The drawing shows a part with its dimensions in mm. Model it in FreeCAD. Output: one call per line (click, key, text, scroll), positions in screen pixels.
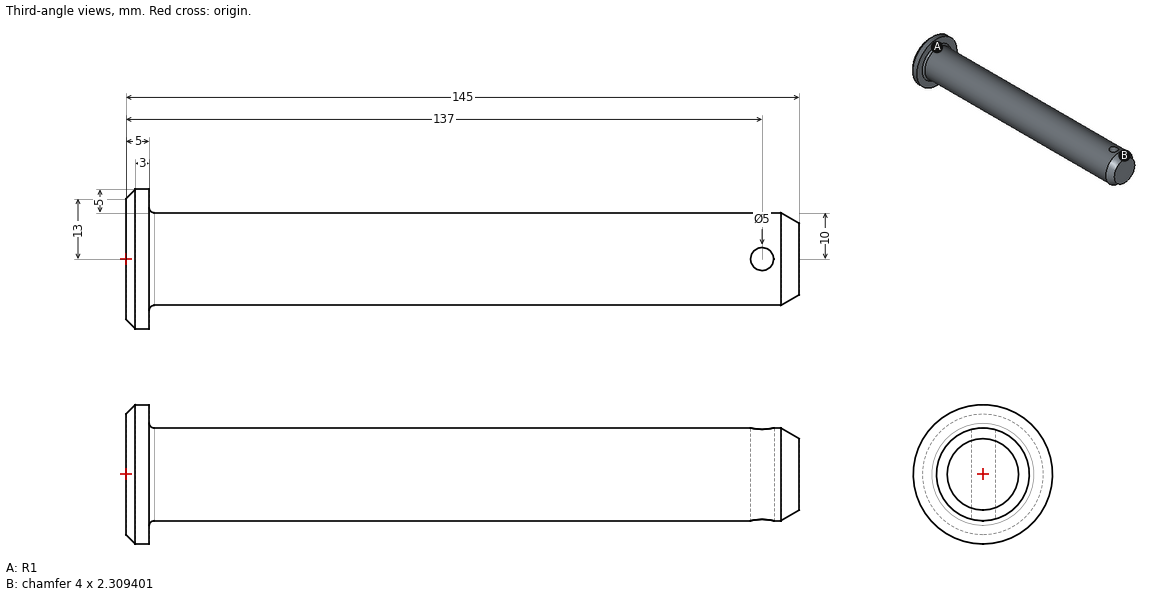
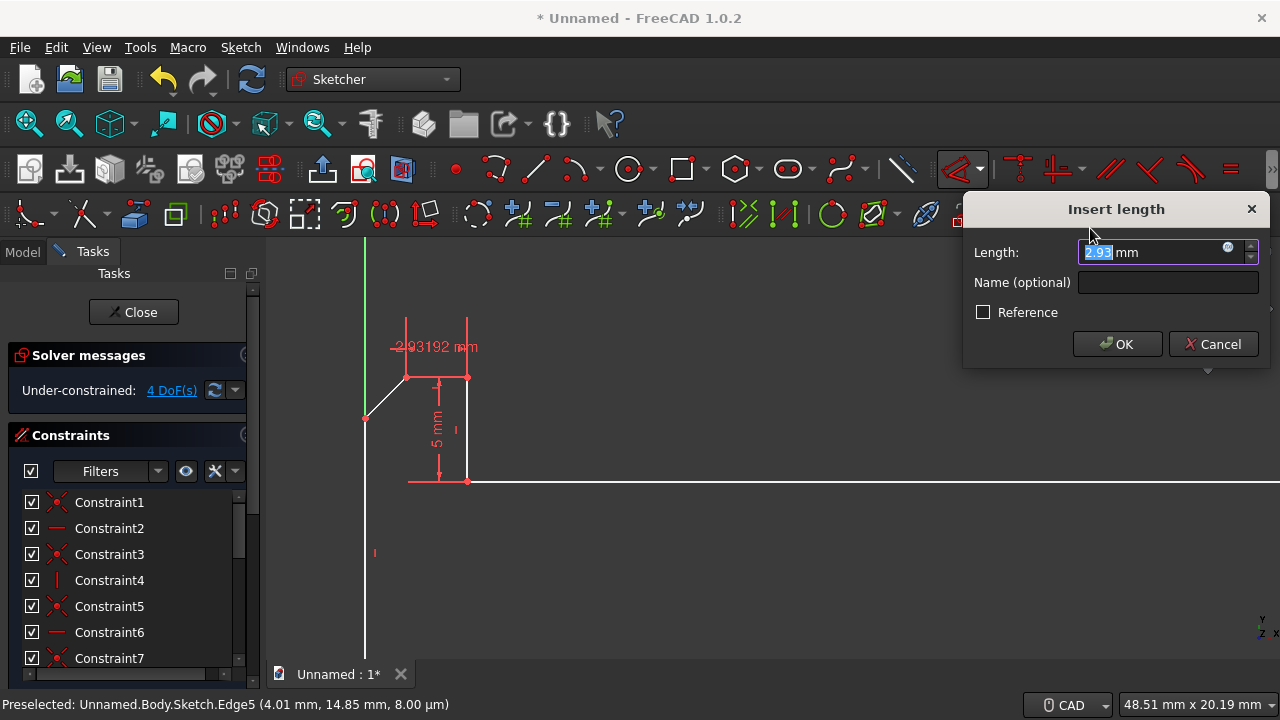
text(3)
key(Return)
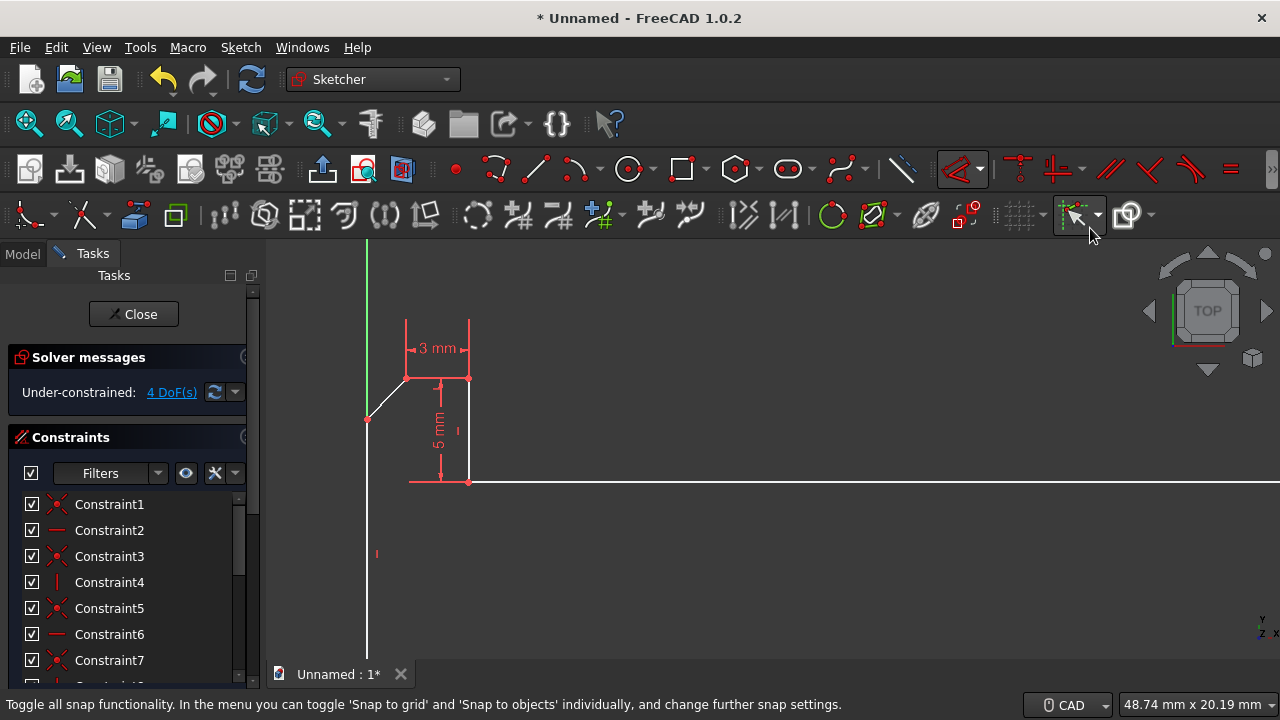
scroll(408, 428, down, 8)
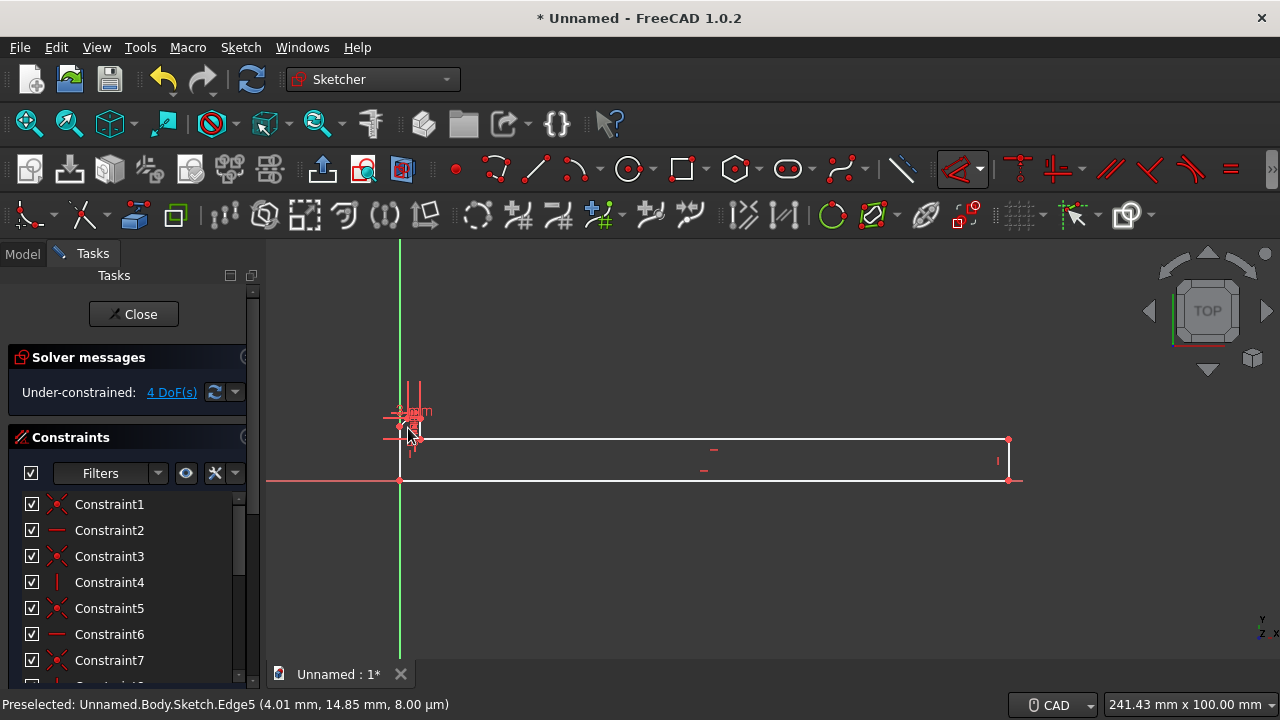
click(1009, 468)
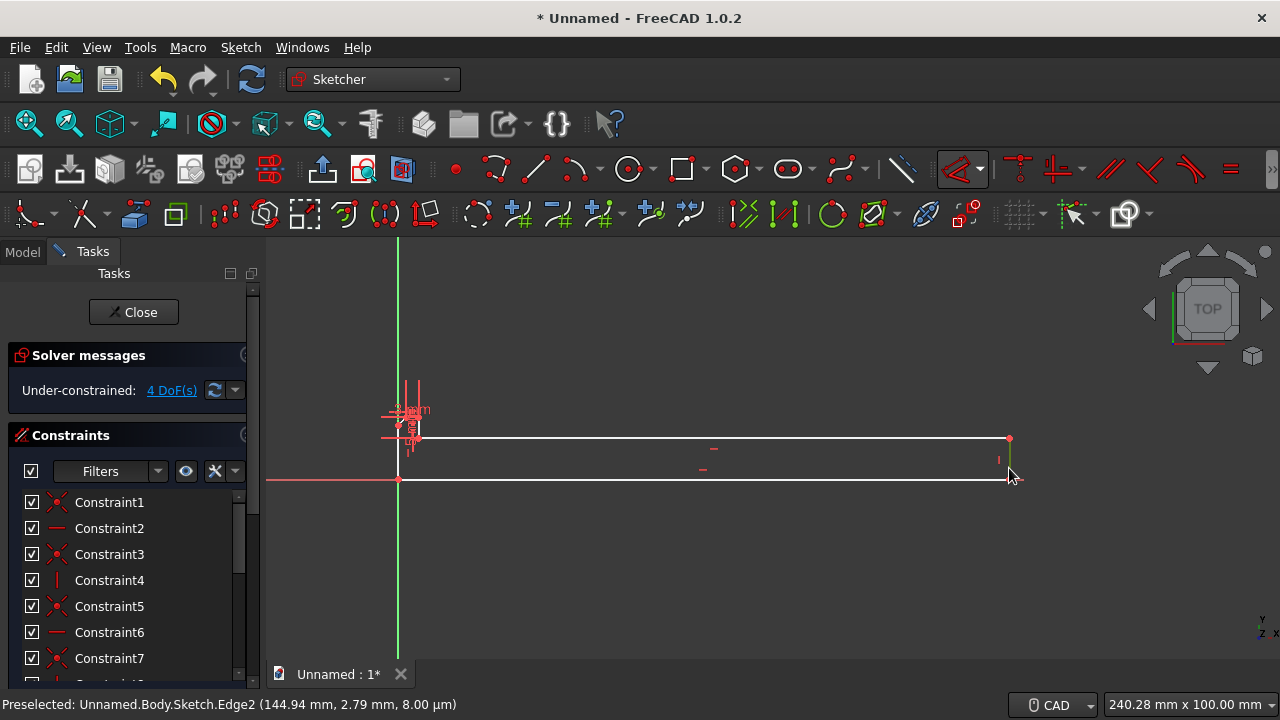
key(i)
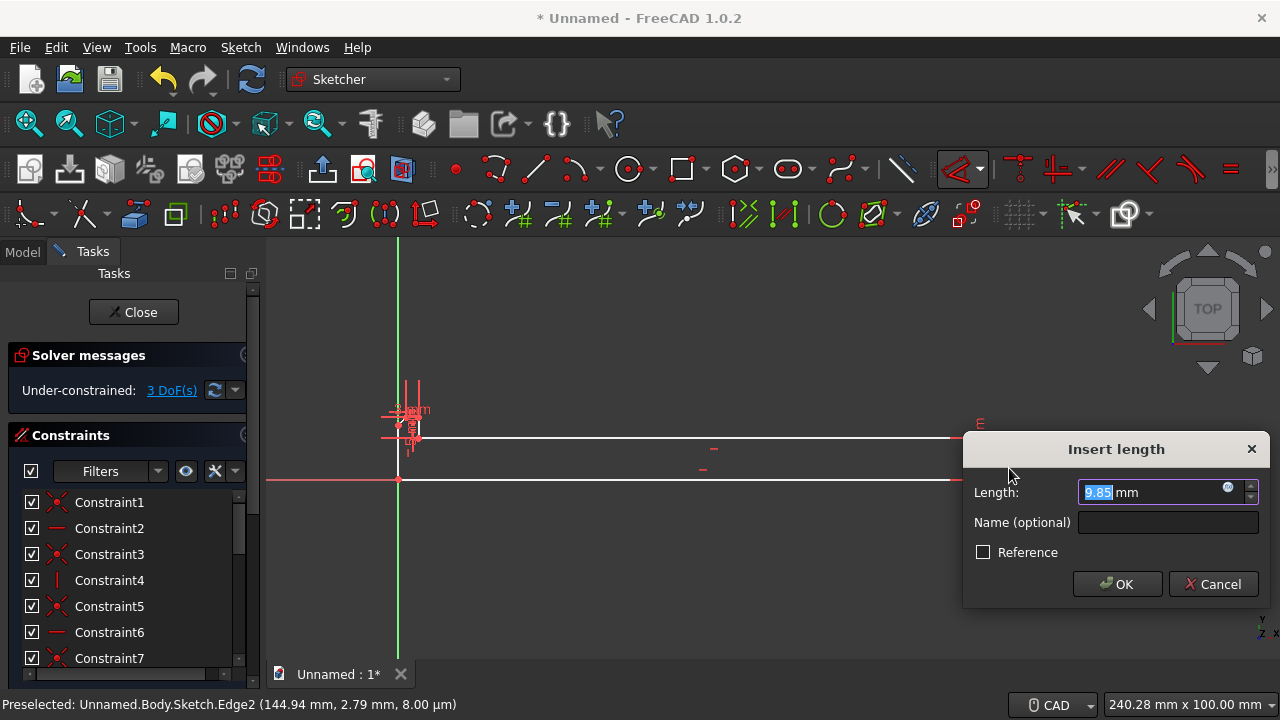
text(10)
key(Return)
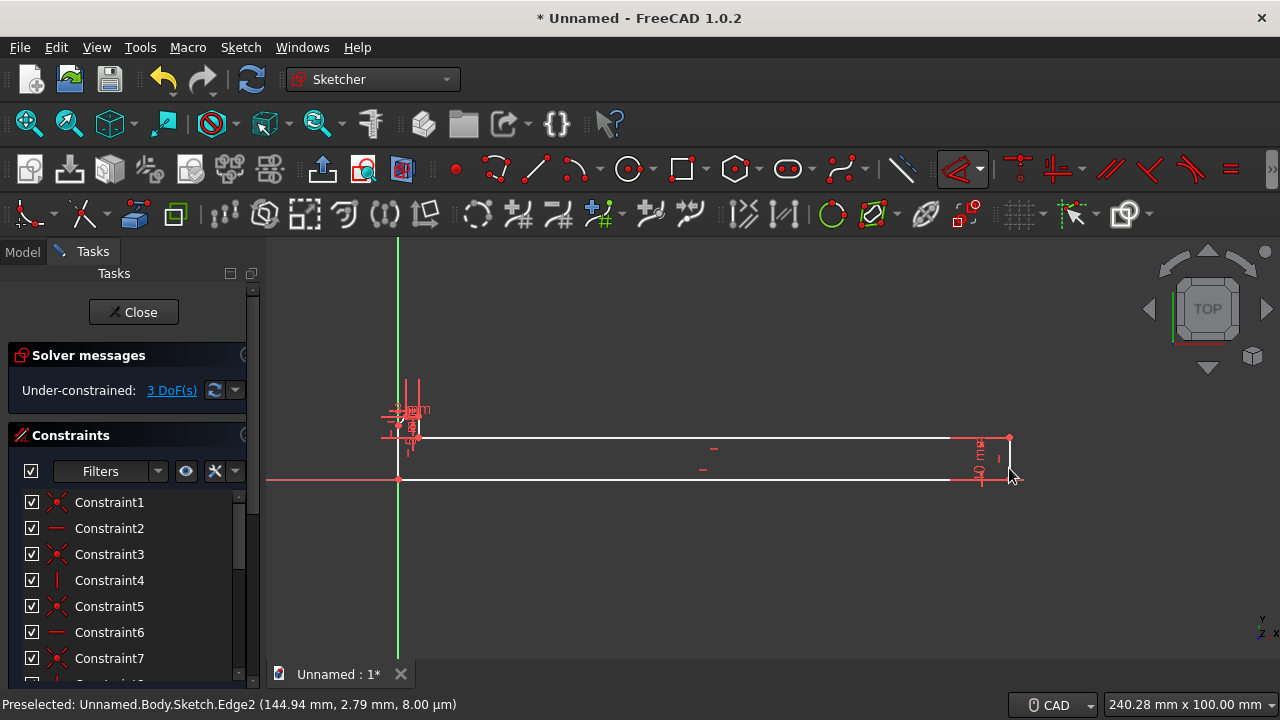
click(398, 442)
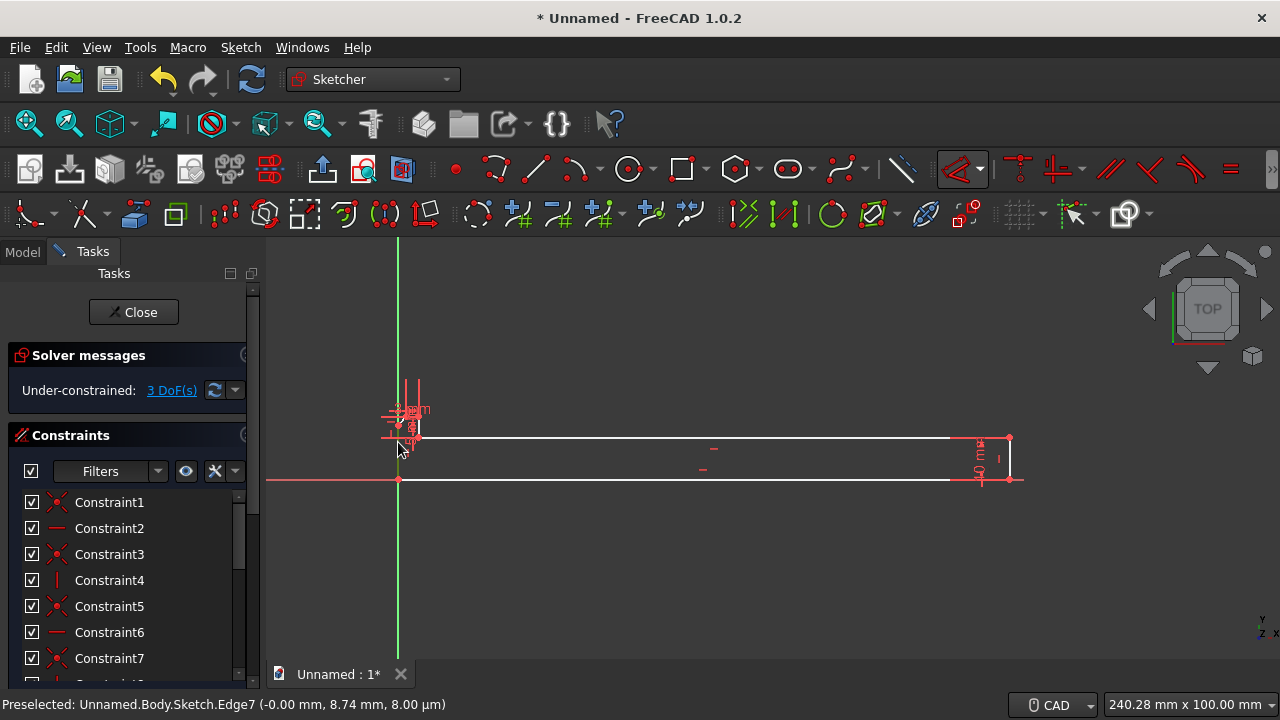
key(i)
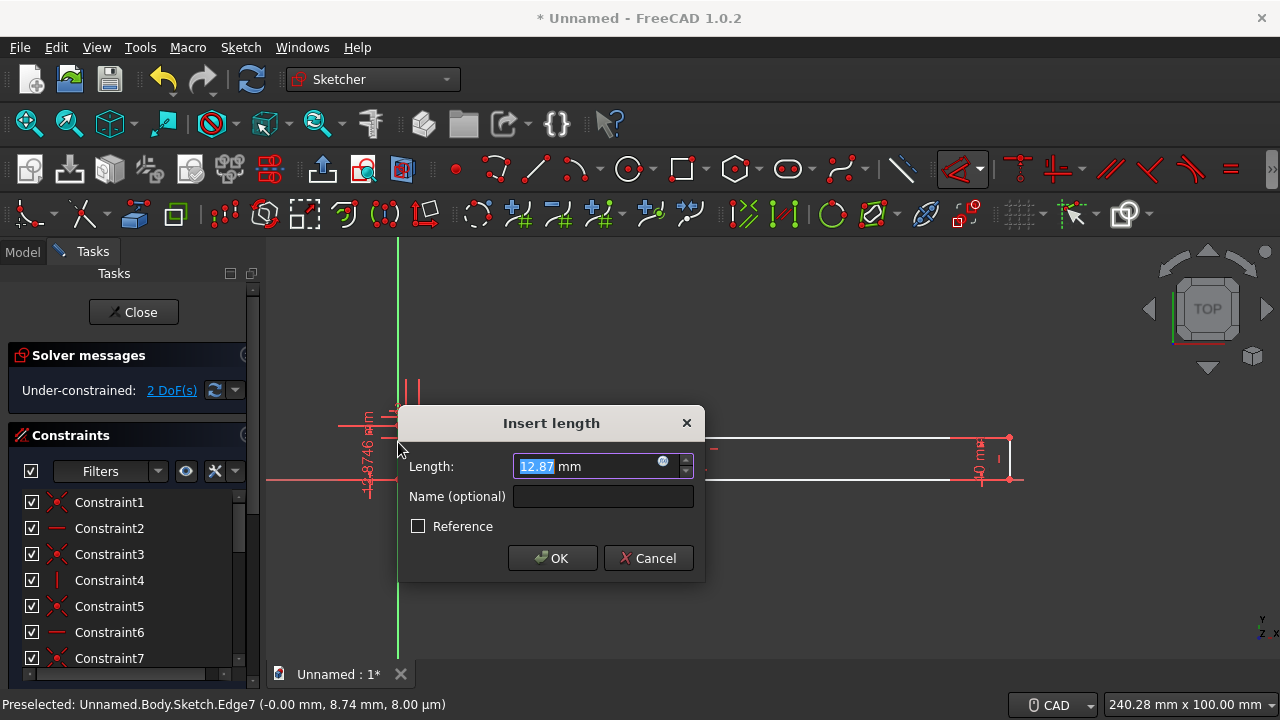
text(13)
key(Return)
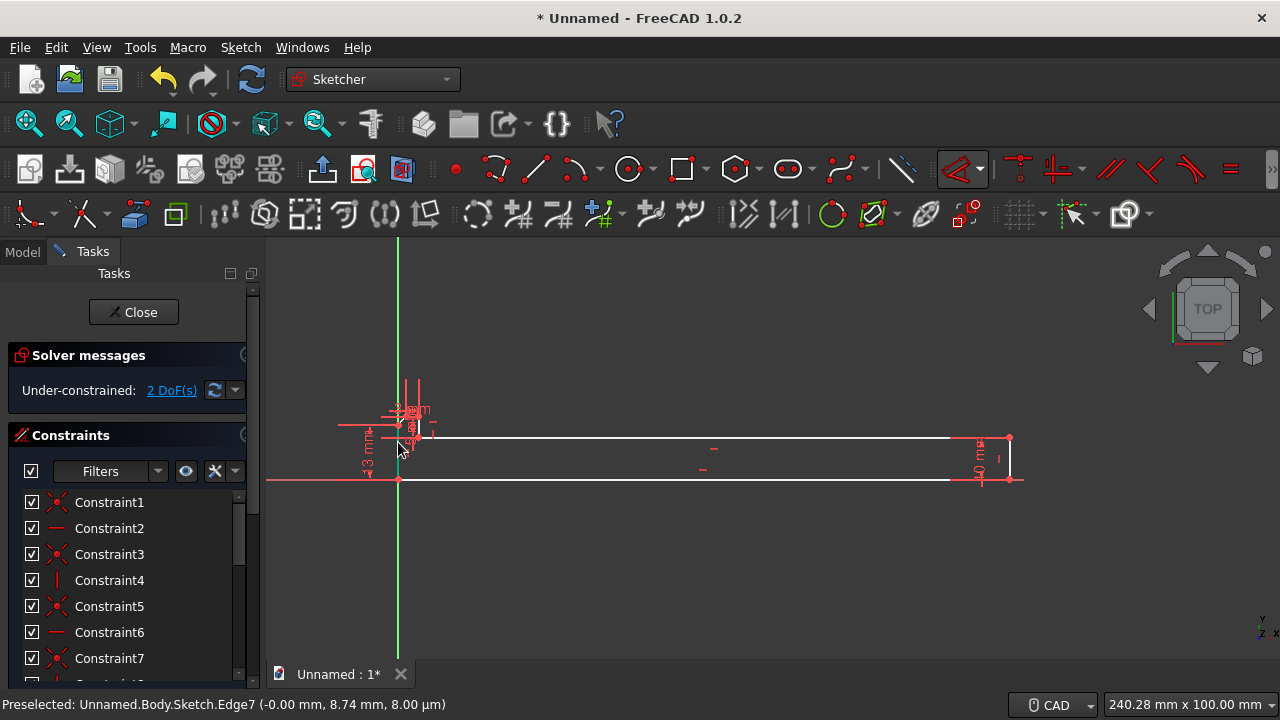
scroll(419, 438, up, 4)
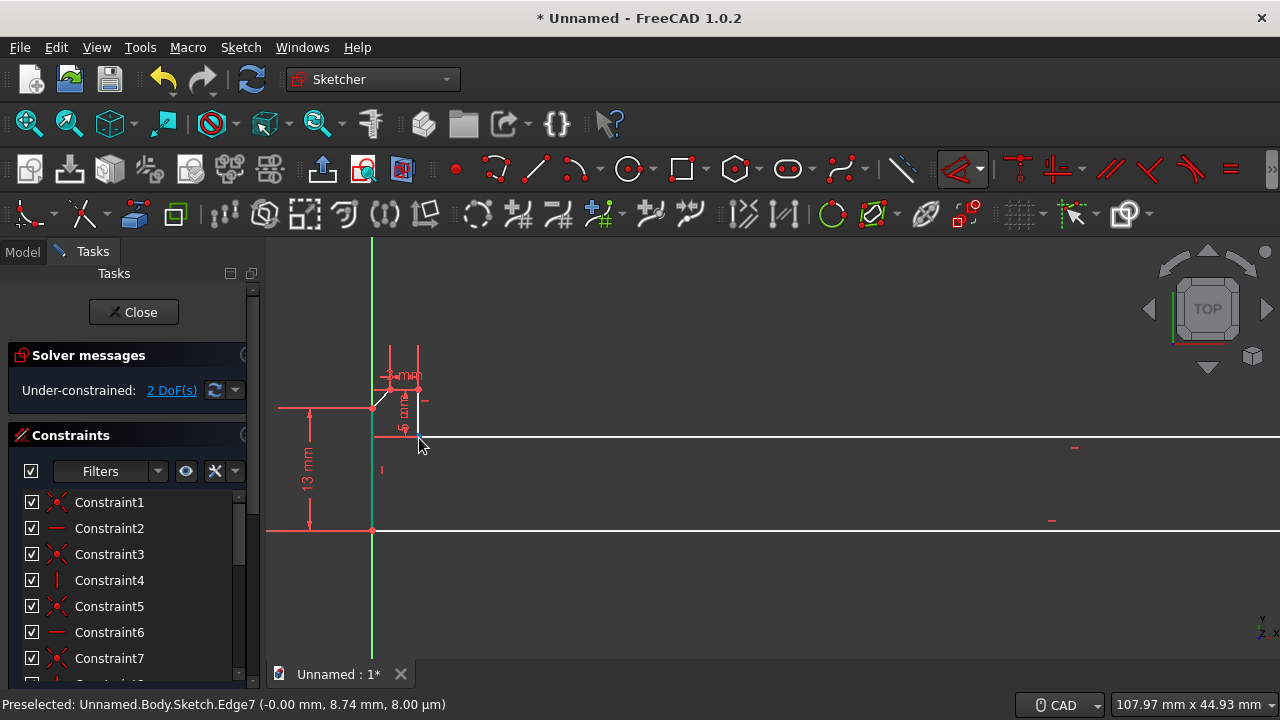
click(418, 437)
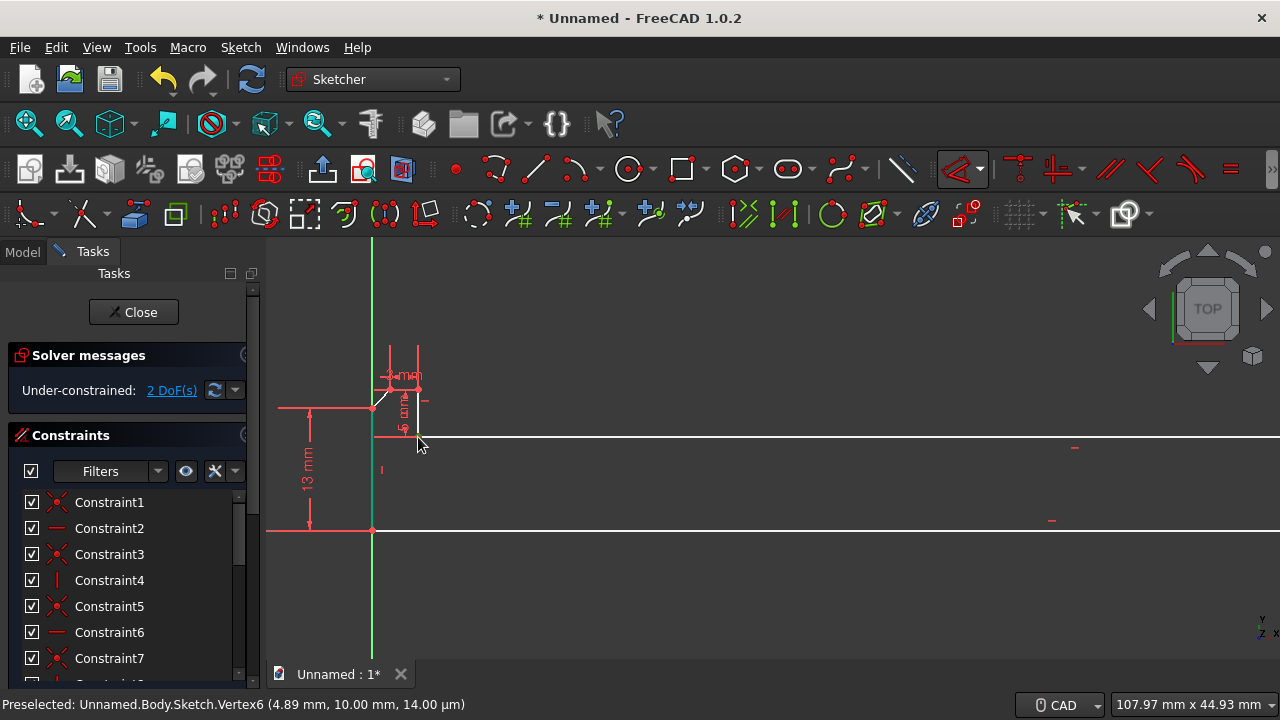
key(l)